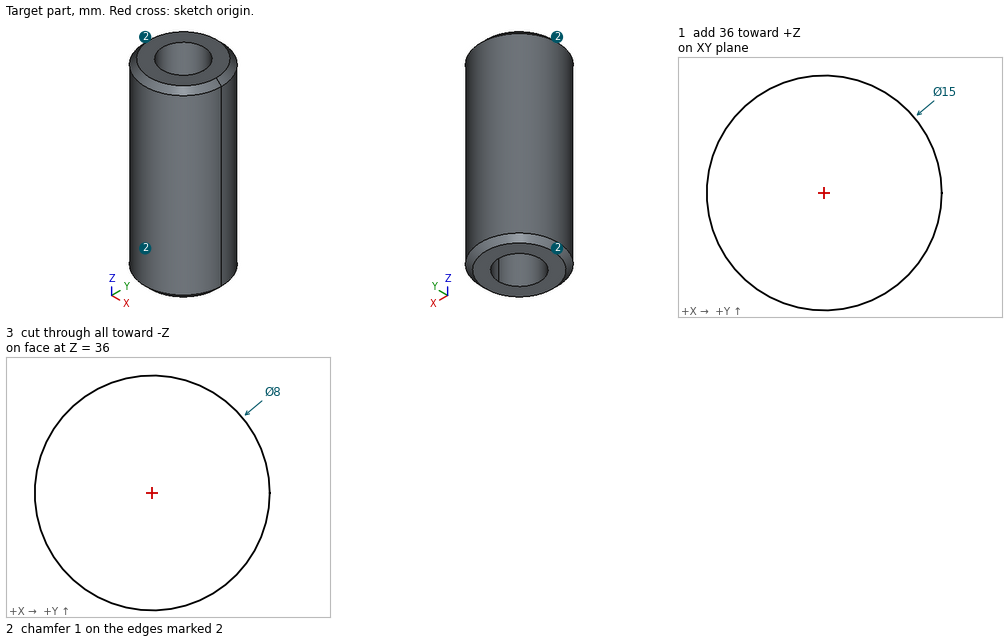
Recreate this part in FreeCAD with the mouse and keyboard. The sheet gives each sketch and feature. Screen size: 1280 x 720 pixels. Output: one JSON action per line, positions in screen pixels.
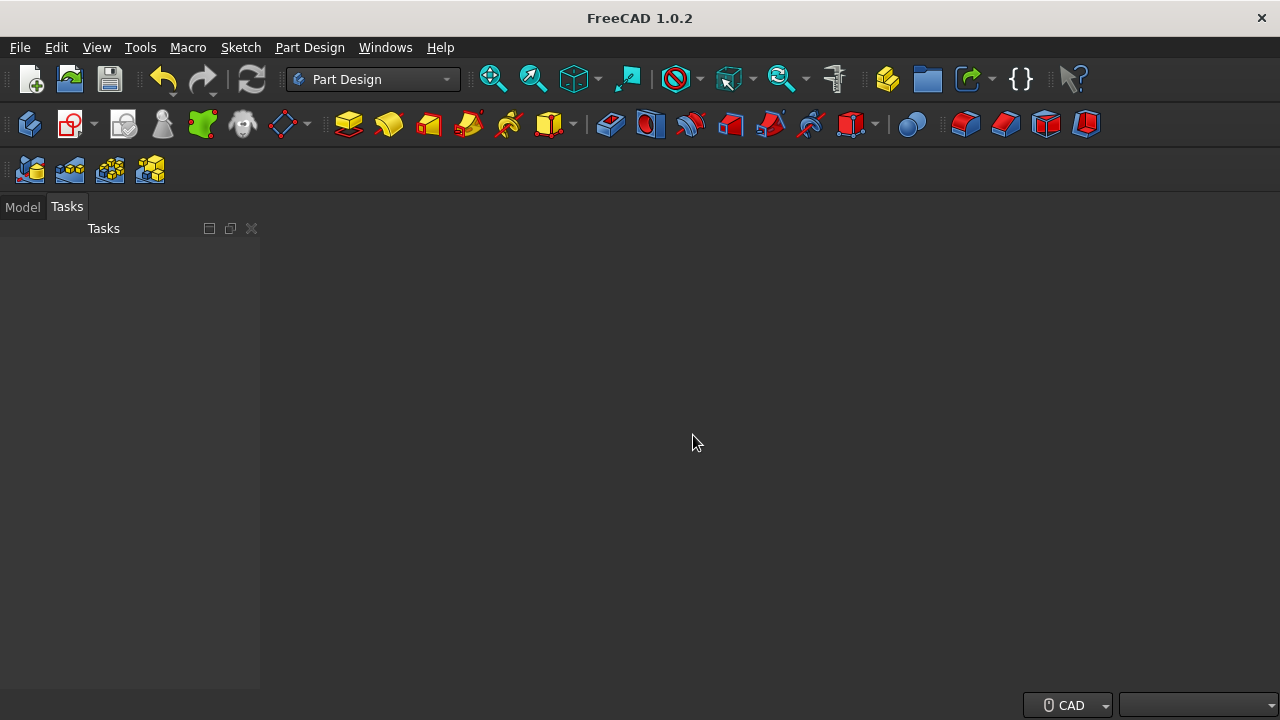
{"action": "left_click", "coordinate": [30, 80]}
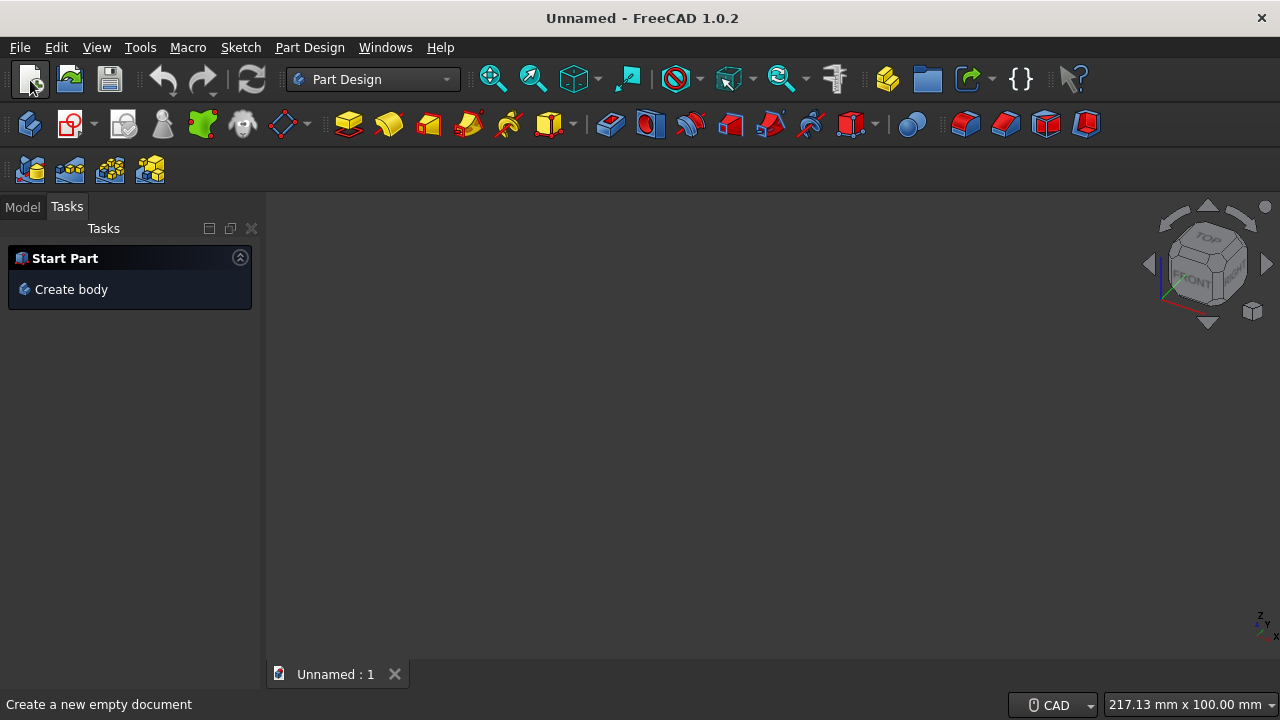
{"action": "left_click", "coordinate": [70, 124]}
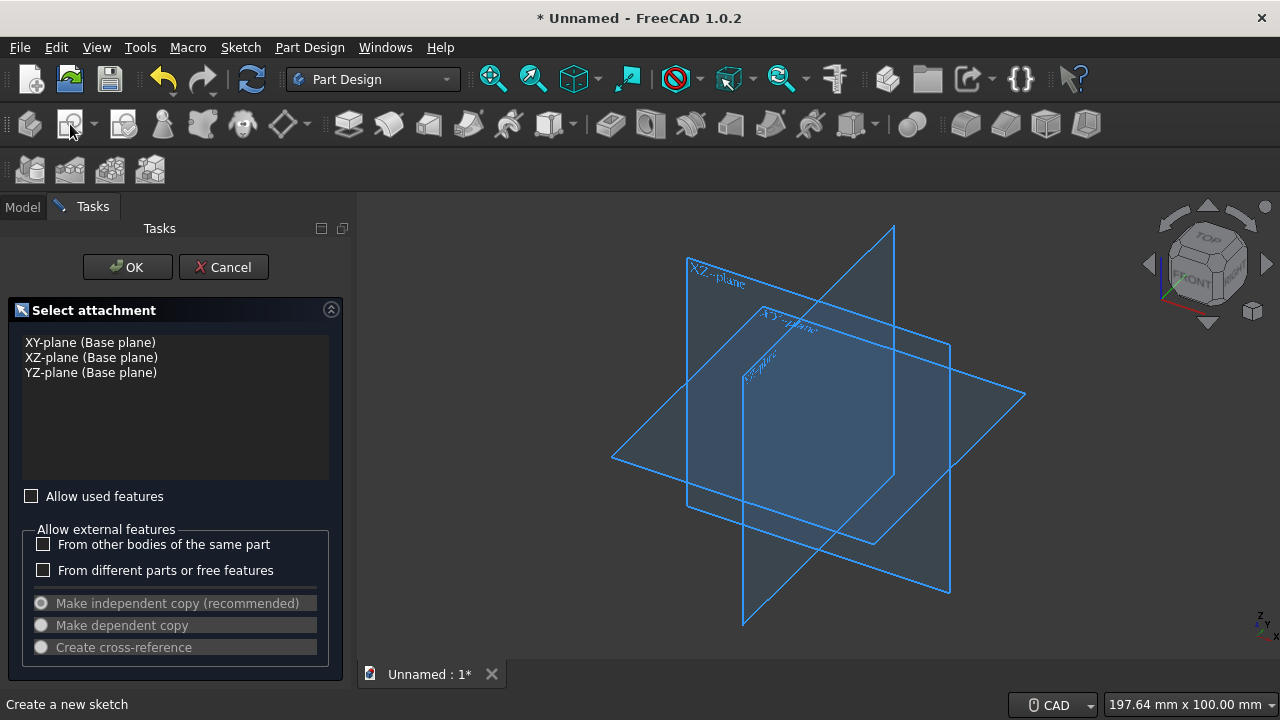
{"action": "left_click", "coordinate": [82, 342]}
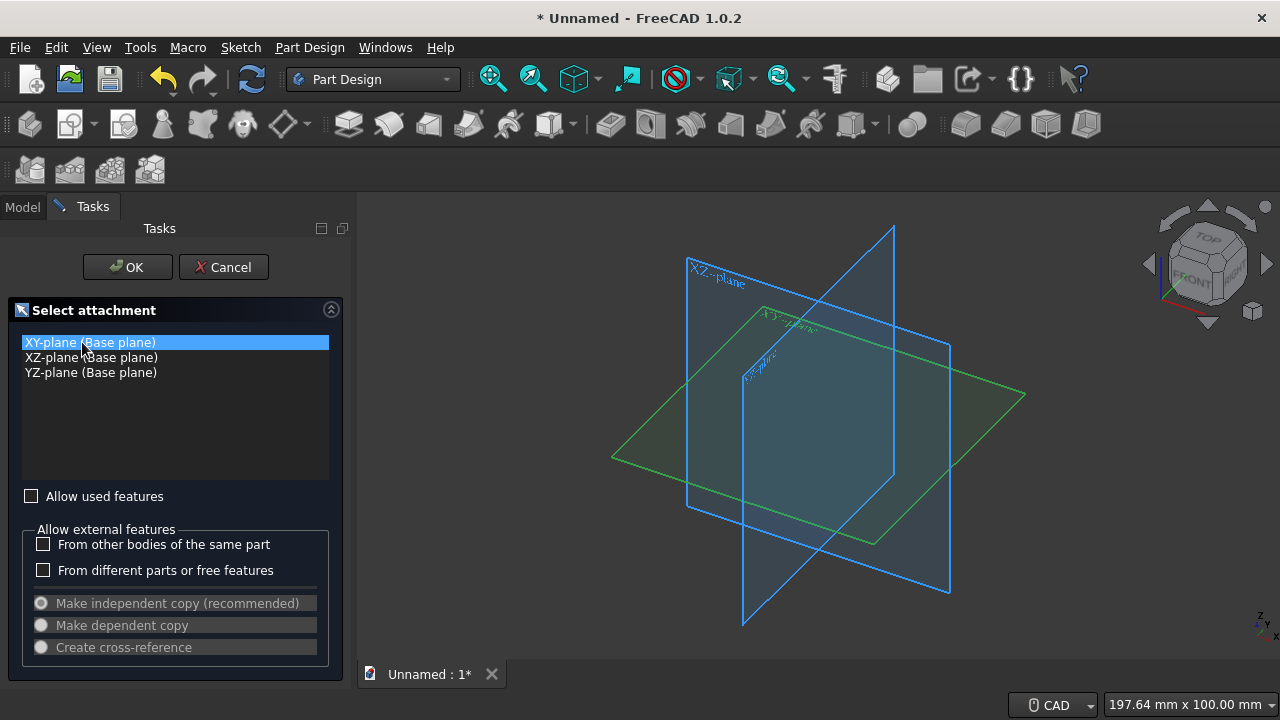
{"action": "left_click", "coordinate": [128, 267]}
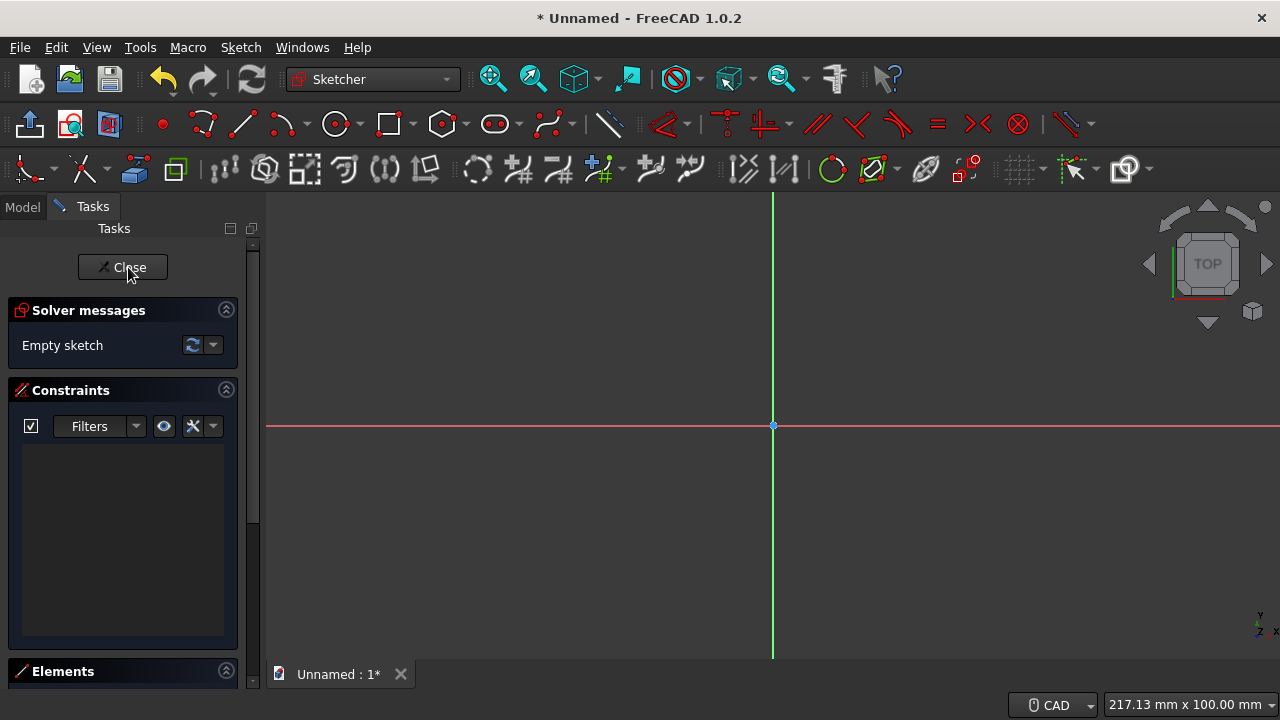
{"action": "scroll", "coordinate": [795, 426], "scroll_direction": "up", "scroll_amount": 7}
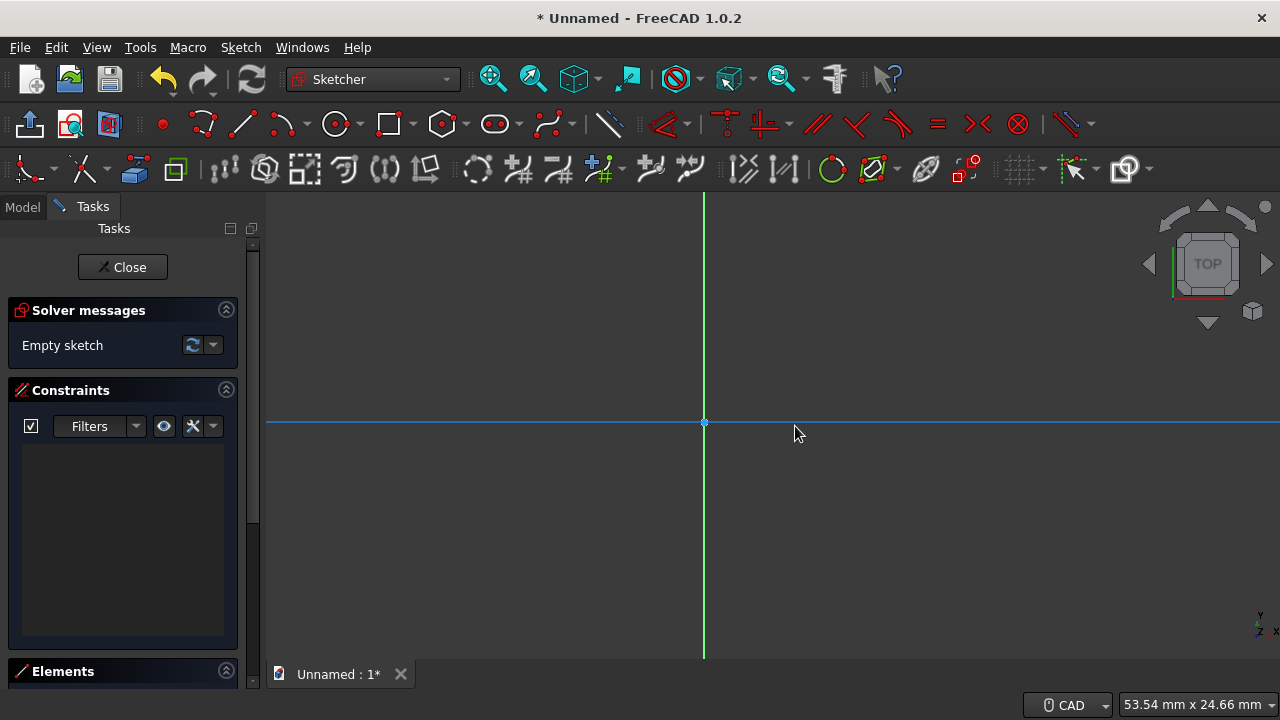
{"action": "left_click", "coordinate": [336, 124]}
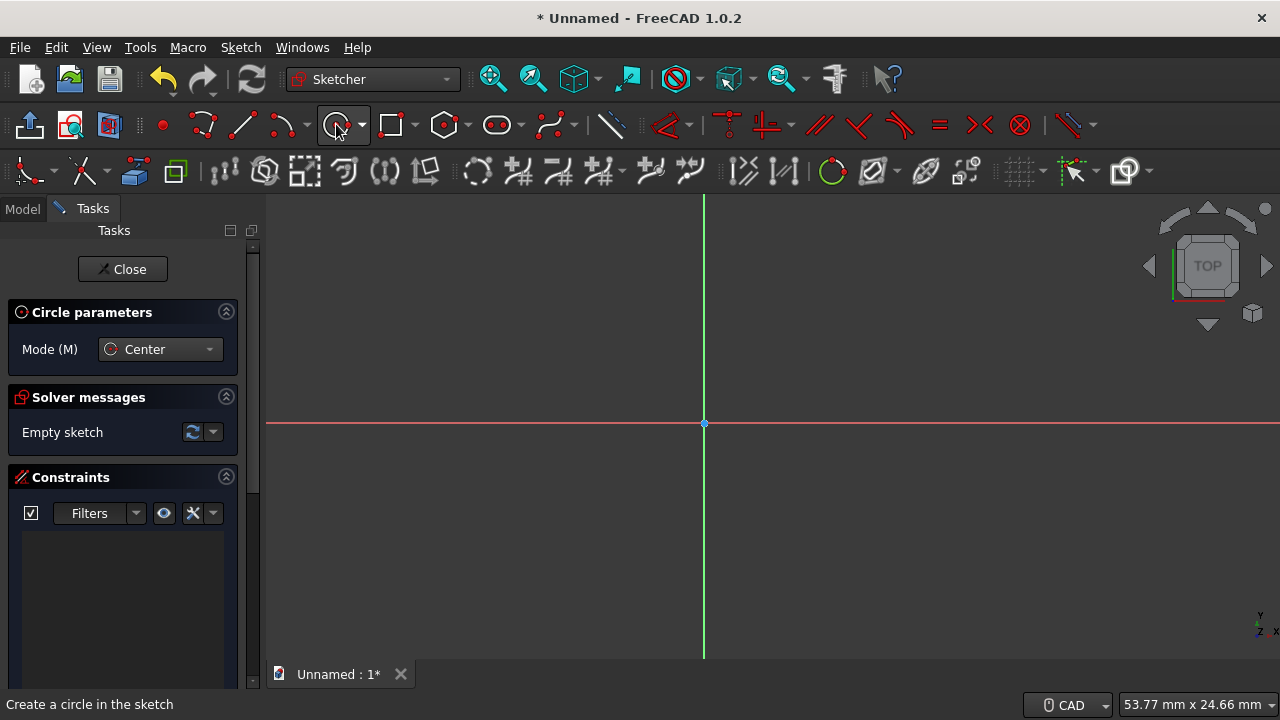
{"action": "left_click", "coordinate": [704, 423]}
{"action": "mouse_move", "coordinate": [804, 323]}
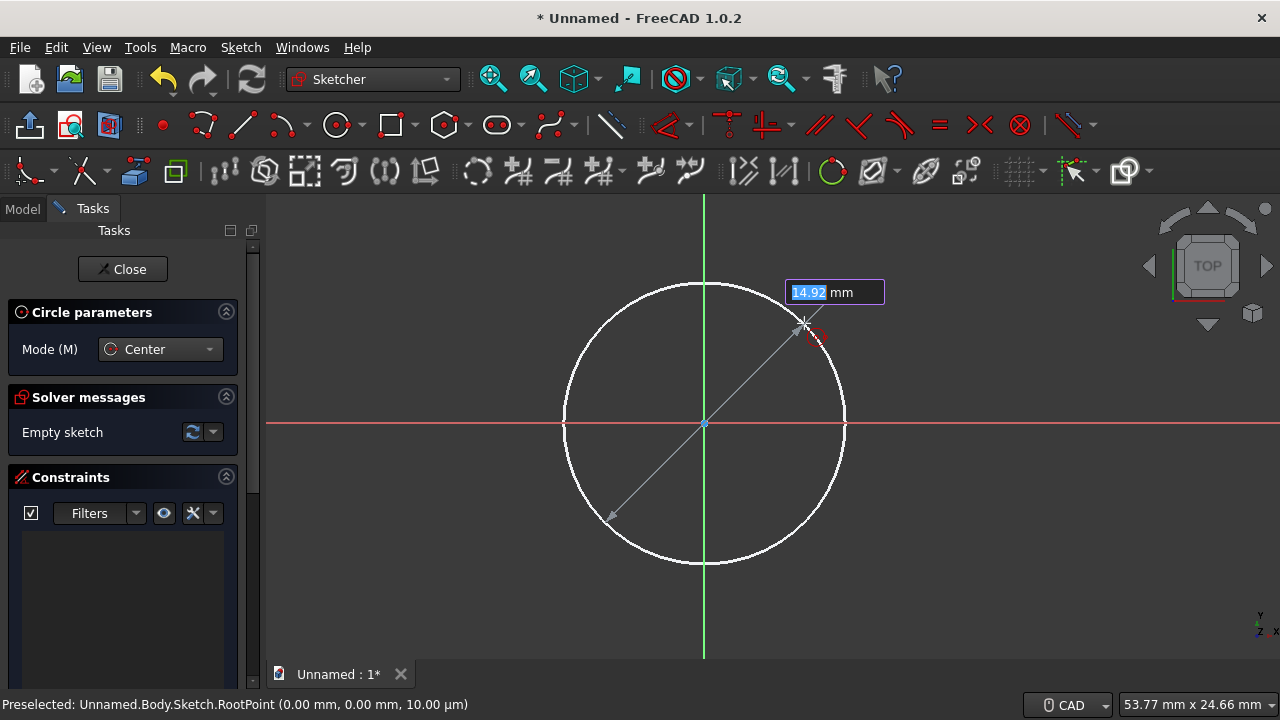
{"action": "type", "text": "15"}
{"action": "key", "text": "Return"}
{"action": "key", "text": "Escape"}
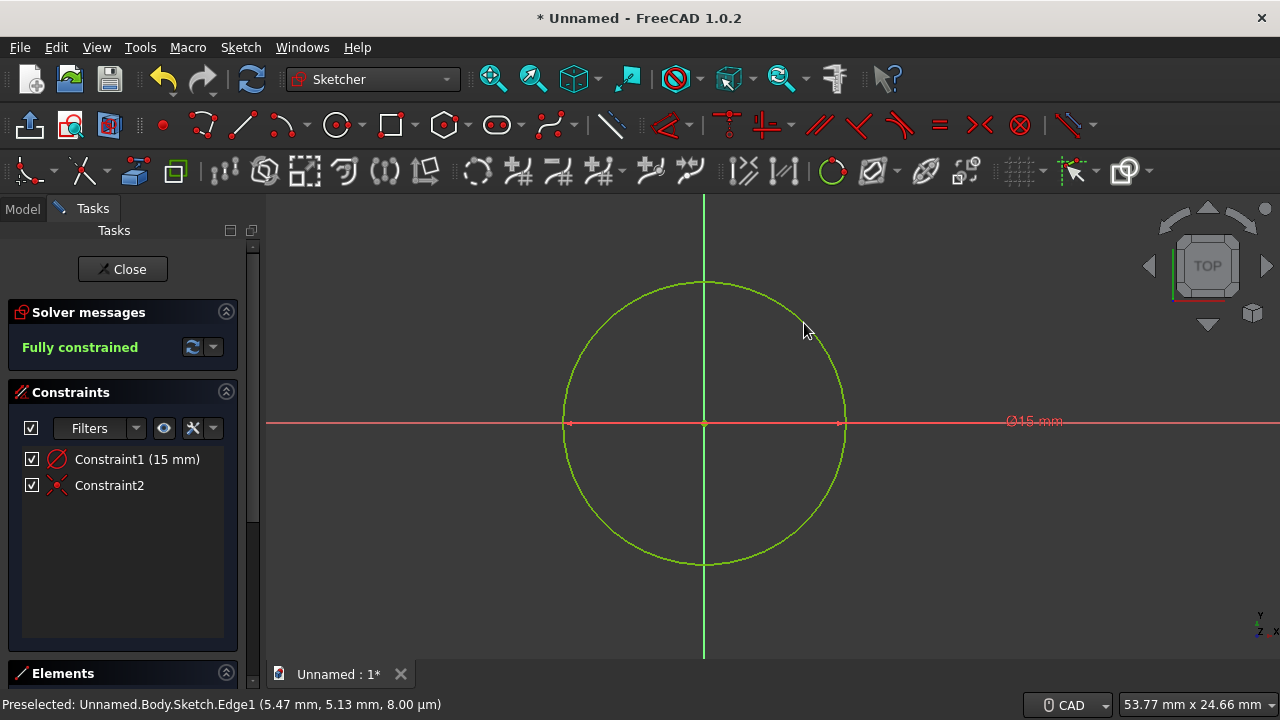
{"action": "left_click", "coordinate": [123, 269]}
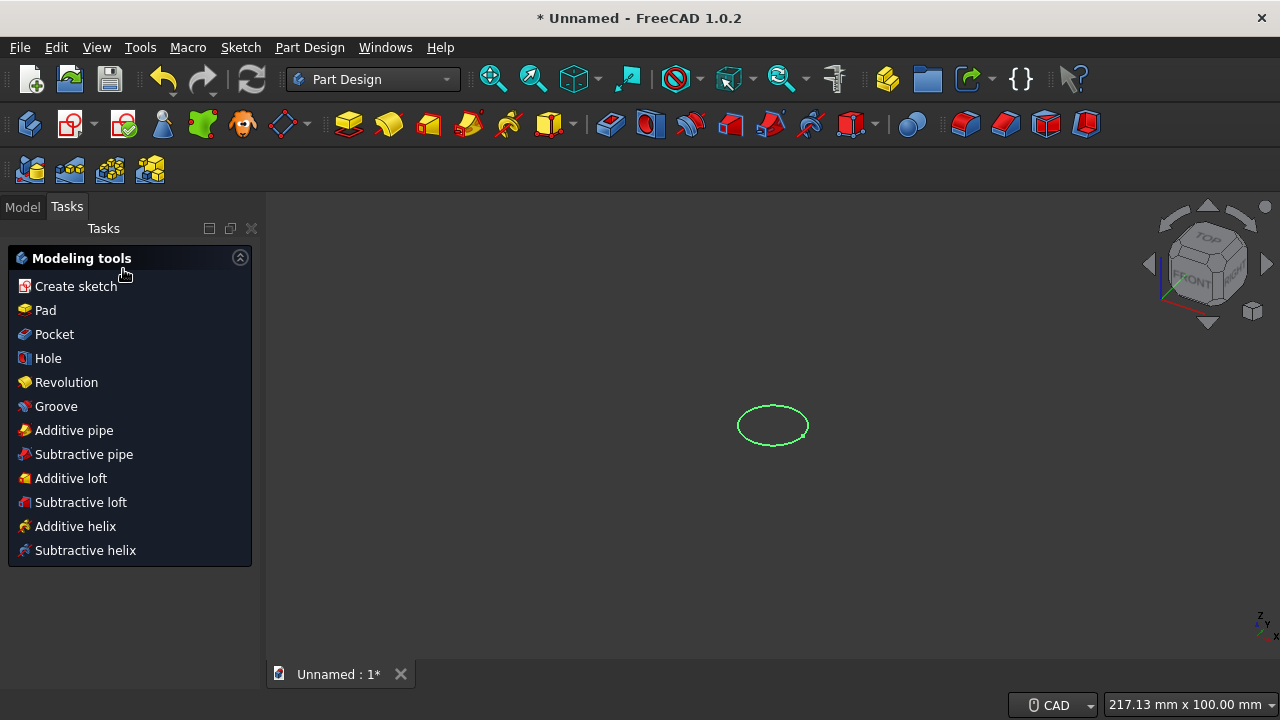
{"action": "left_click", "coordinate": [350, 124]}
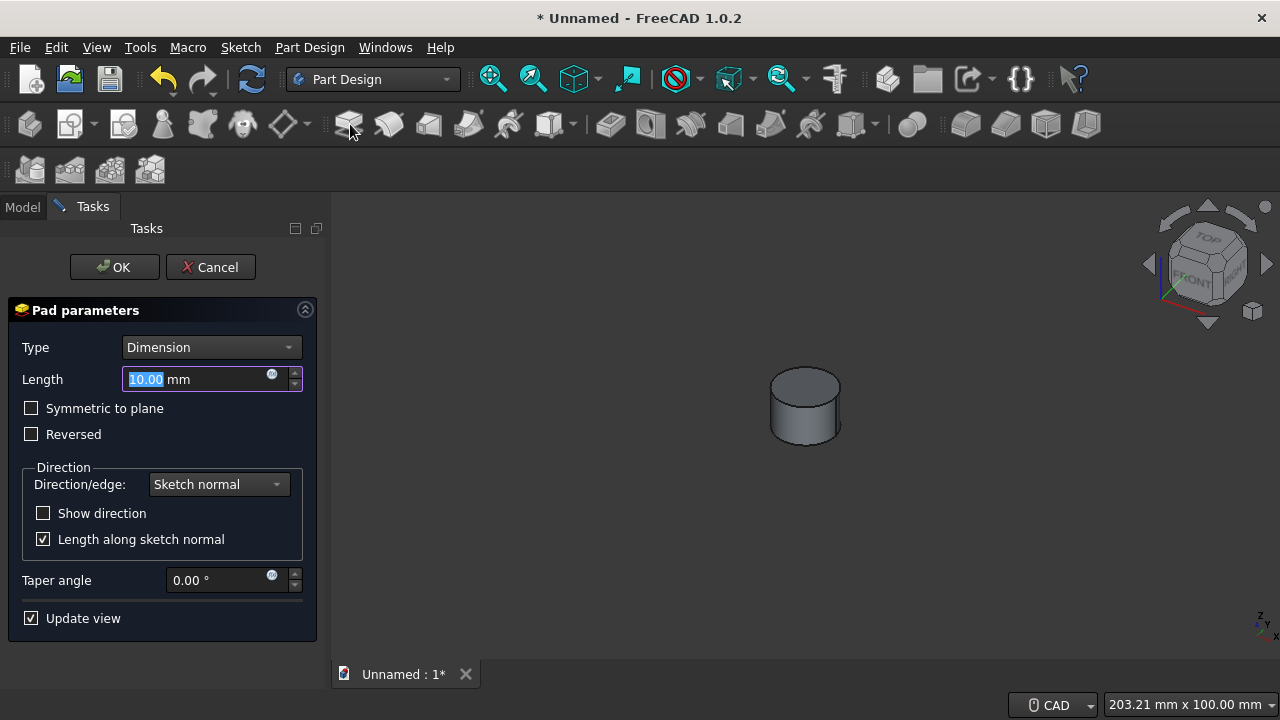
{"action": "type", "text": "36"}
{"action": "key", "text": "Tab"}